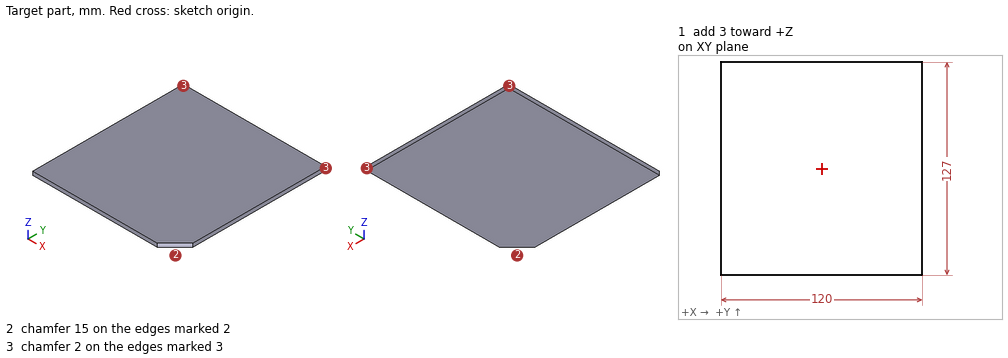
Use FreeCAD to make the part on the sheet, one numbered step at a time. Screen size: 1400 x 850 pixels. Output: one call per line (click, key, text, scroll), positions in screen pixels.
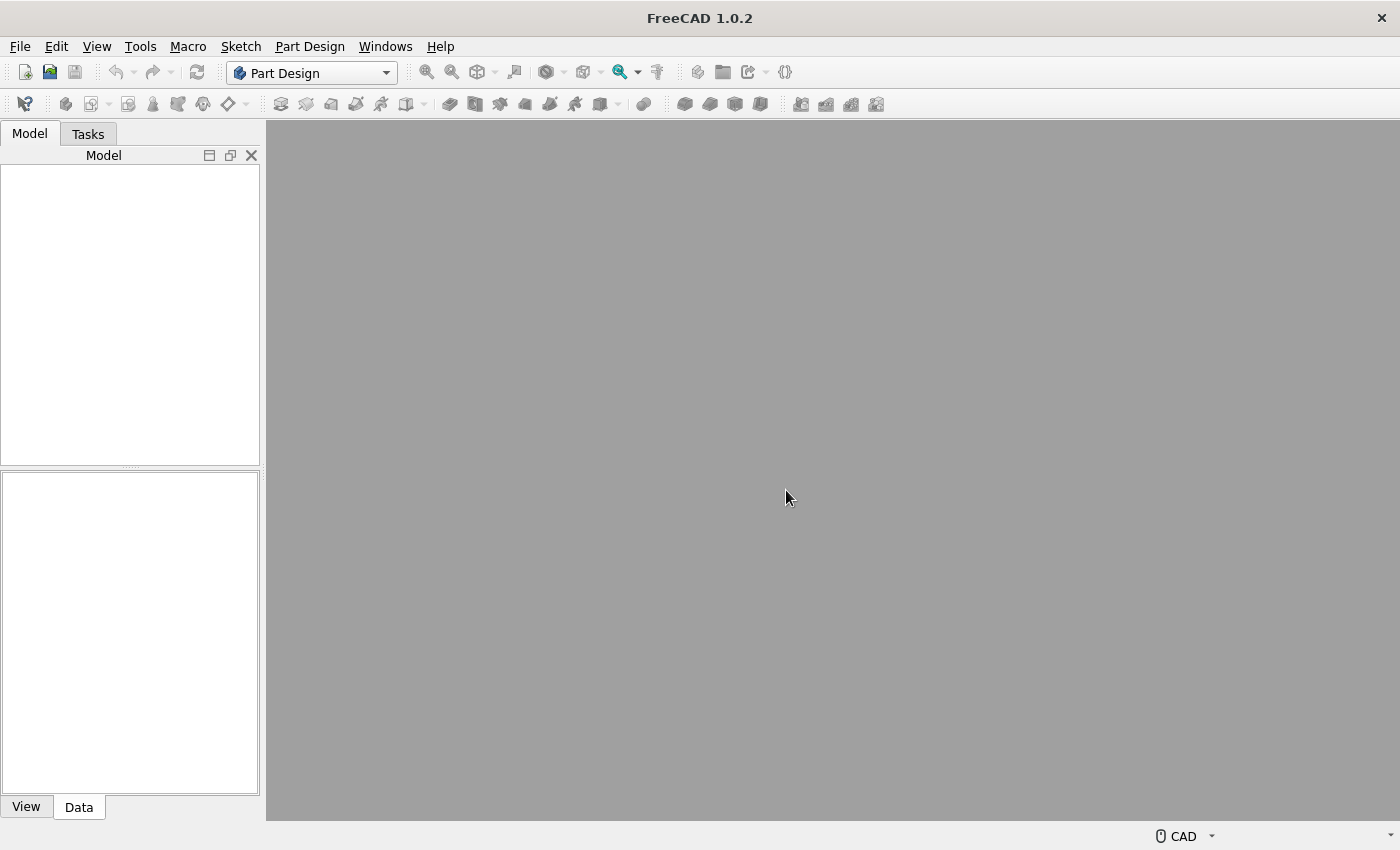
key(ctrl+n)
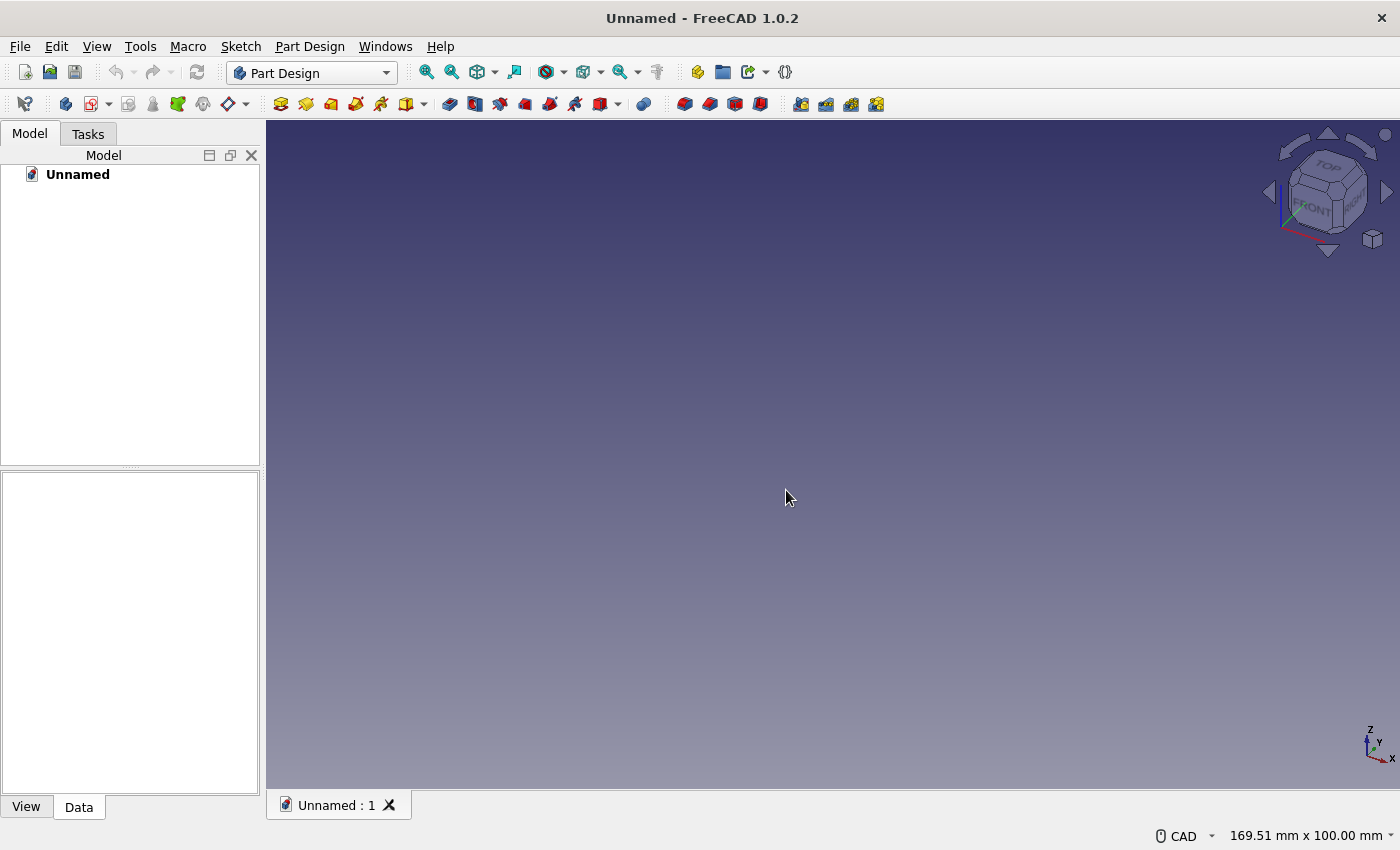
click(90, 104)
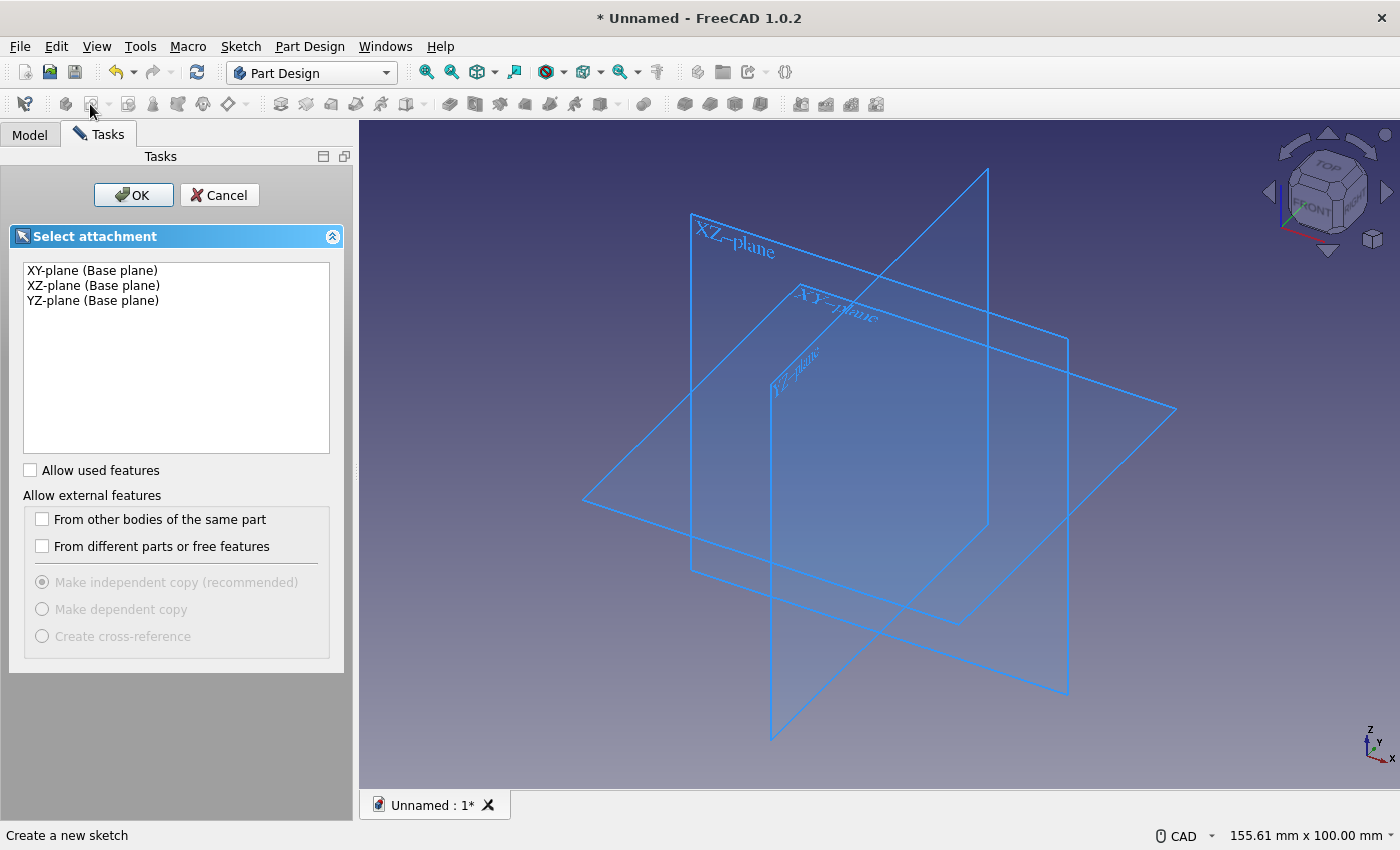
click(84, 270)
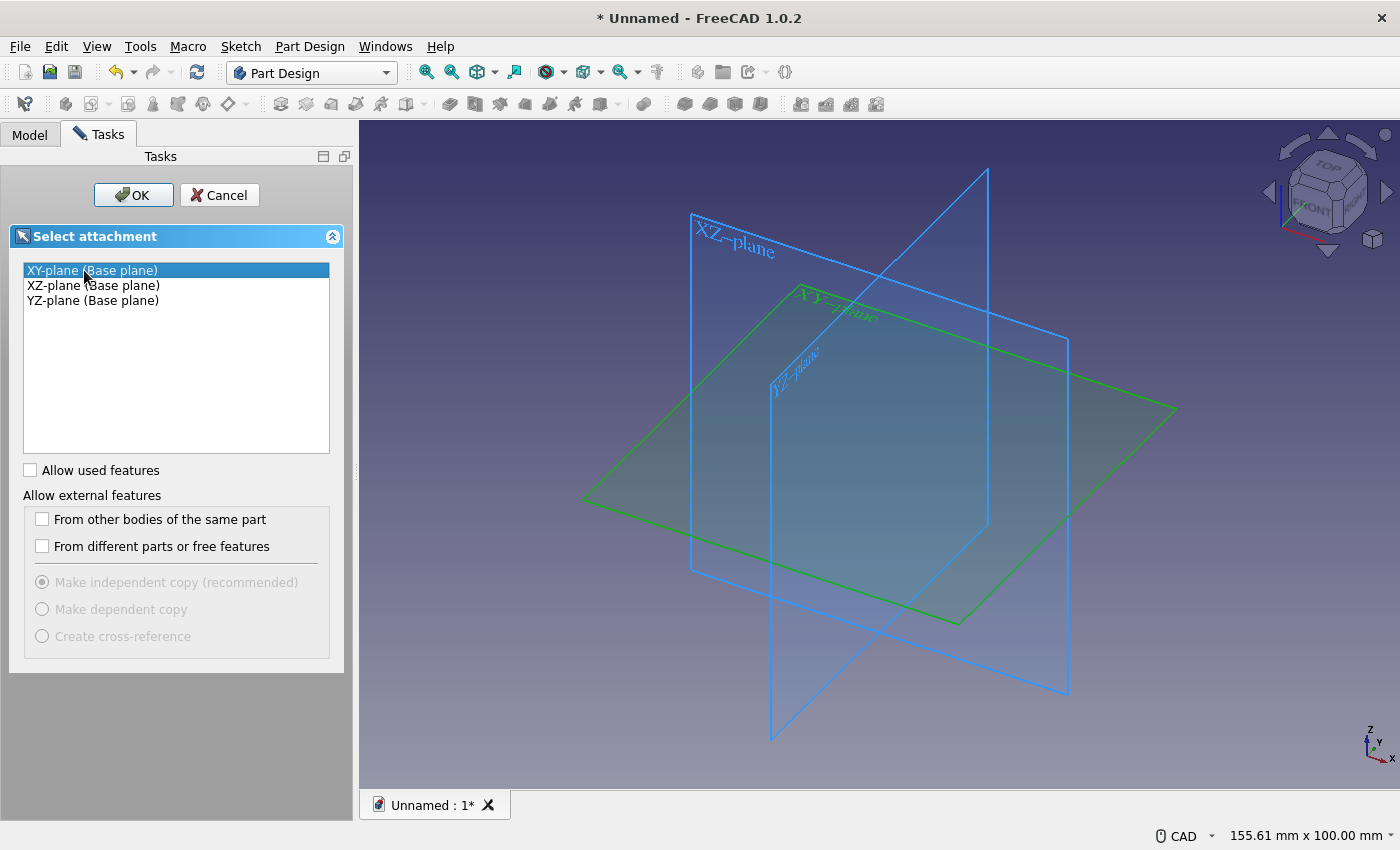
click(134, 195)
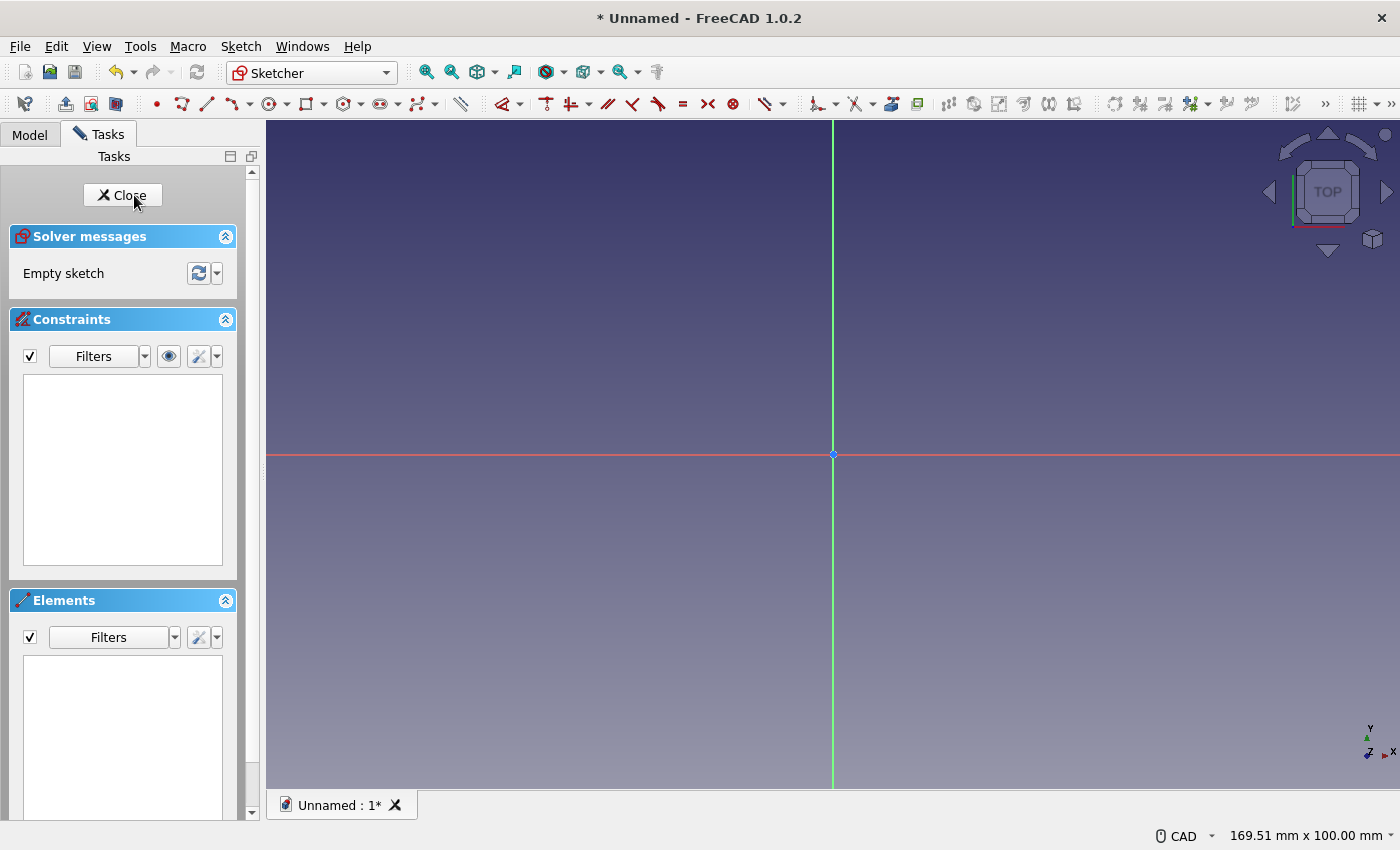
scroll(681, 454, down, 3)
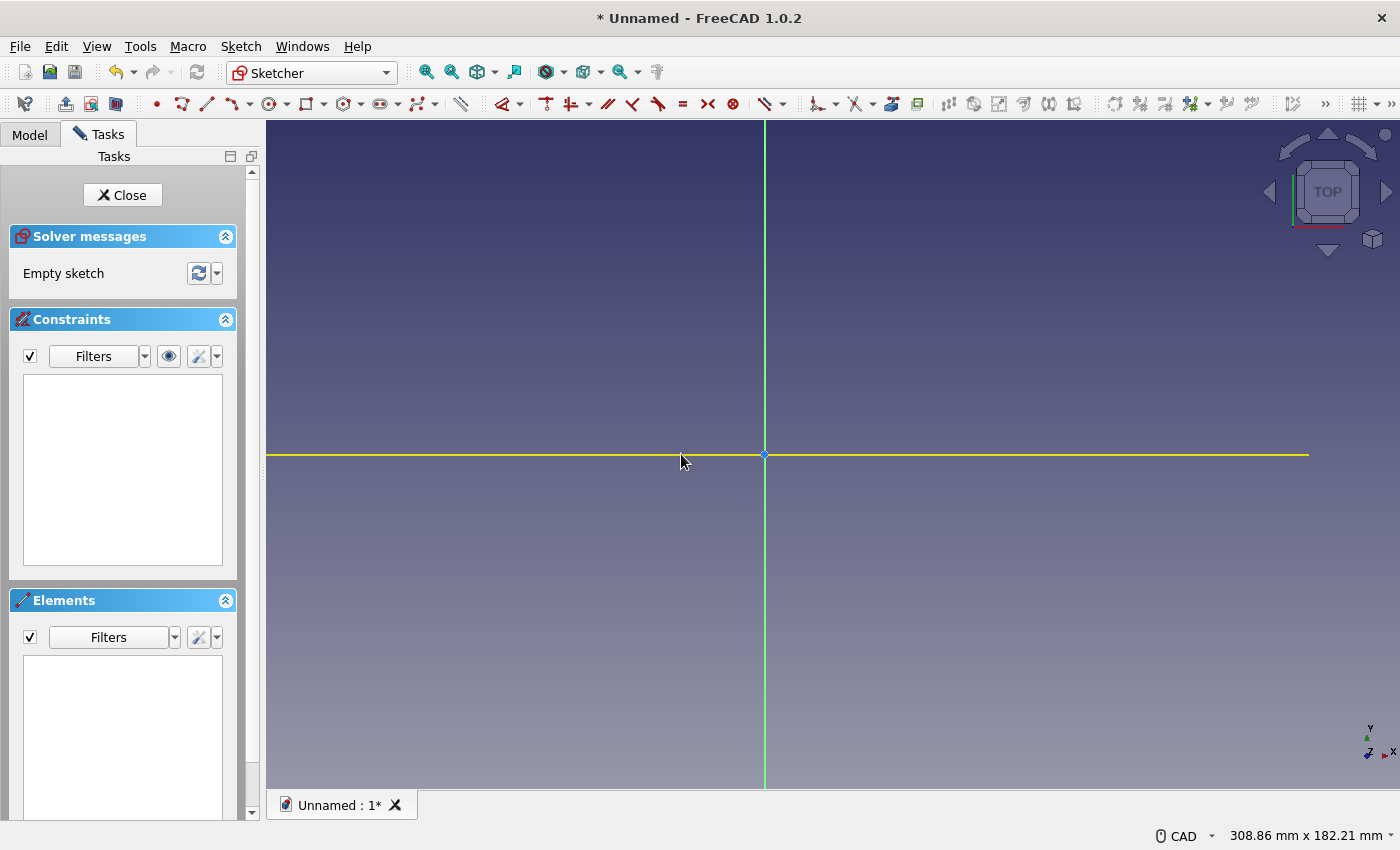
click(324, 104)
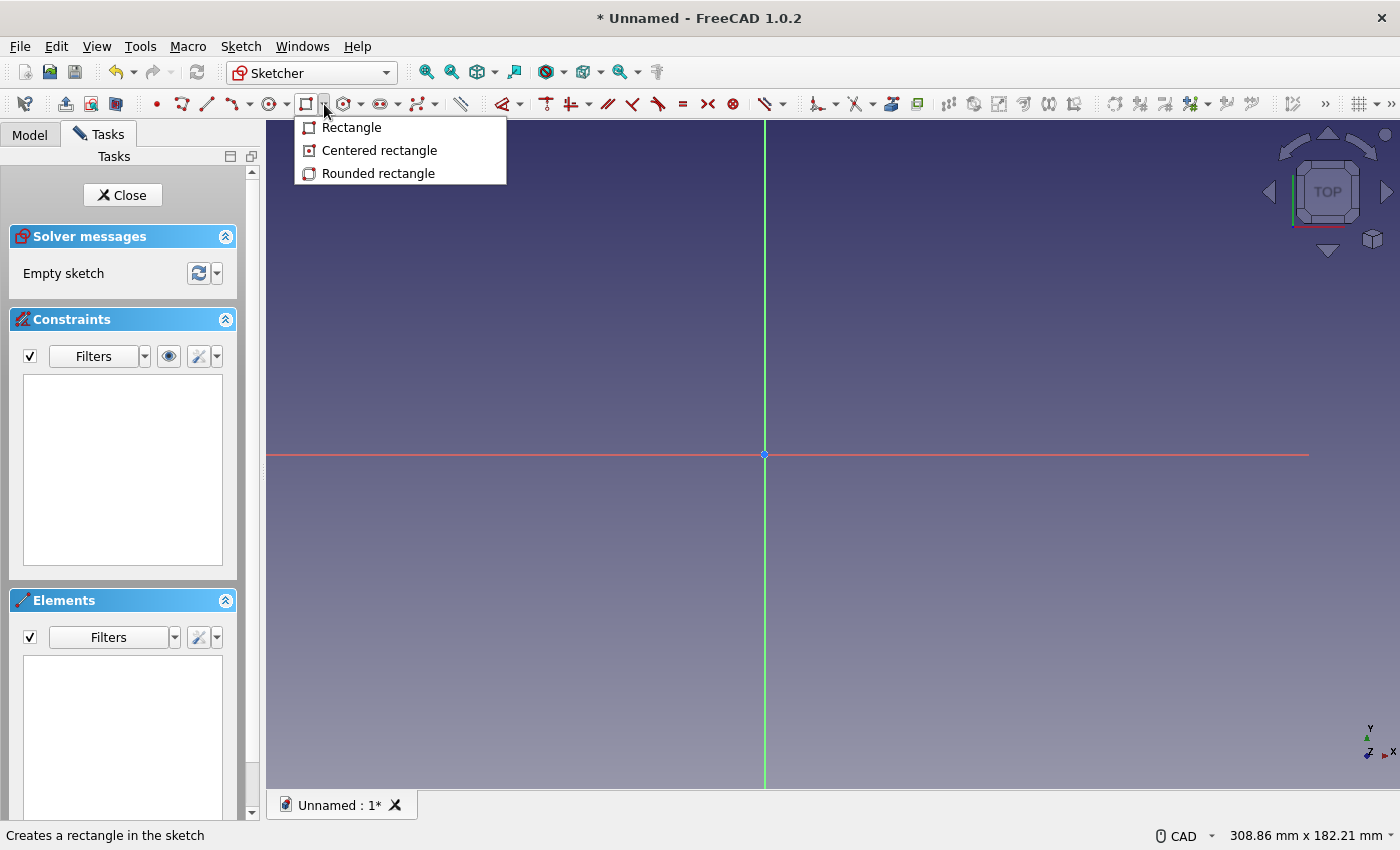
click(400, 150)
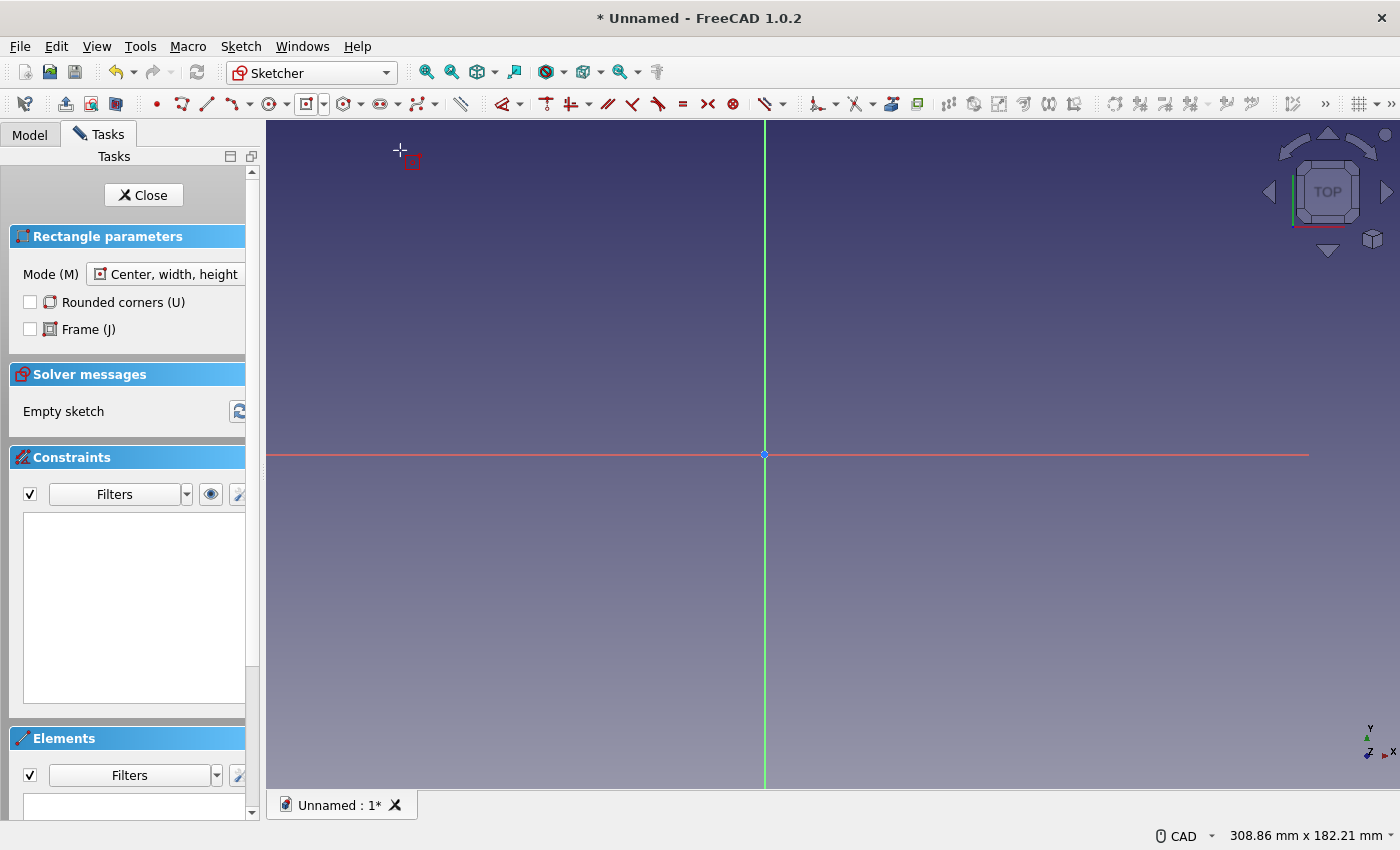
click(765, 454)
click(985, 221)
key(Escape)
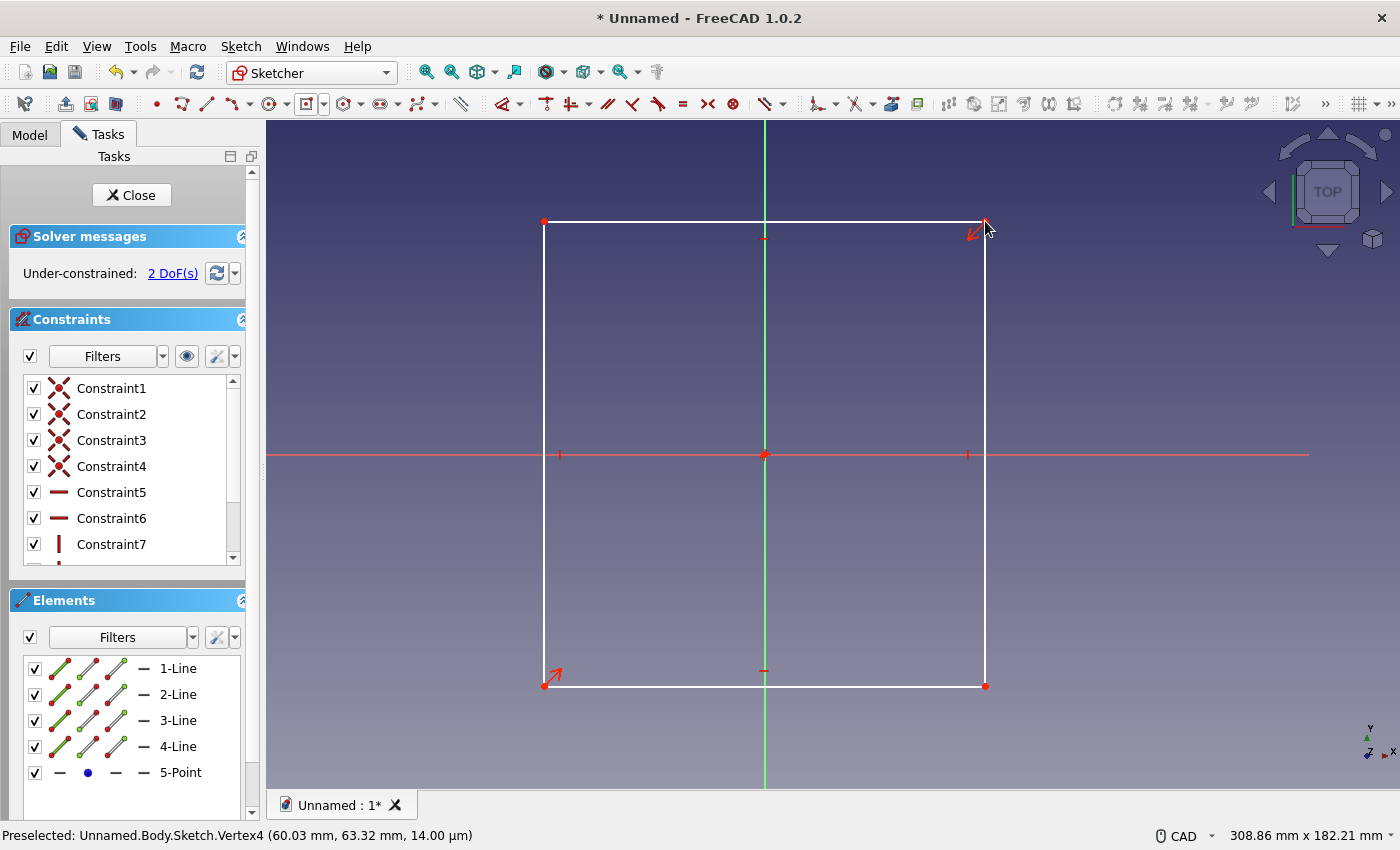
click(676, 687)